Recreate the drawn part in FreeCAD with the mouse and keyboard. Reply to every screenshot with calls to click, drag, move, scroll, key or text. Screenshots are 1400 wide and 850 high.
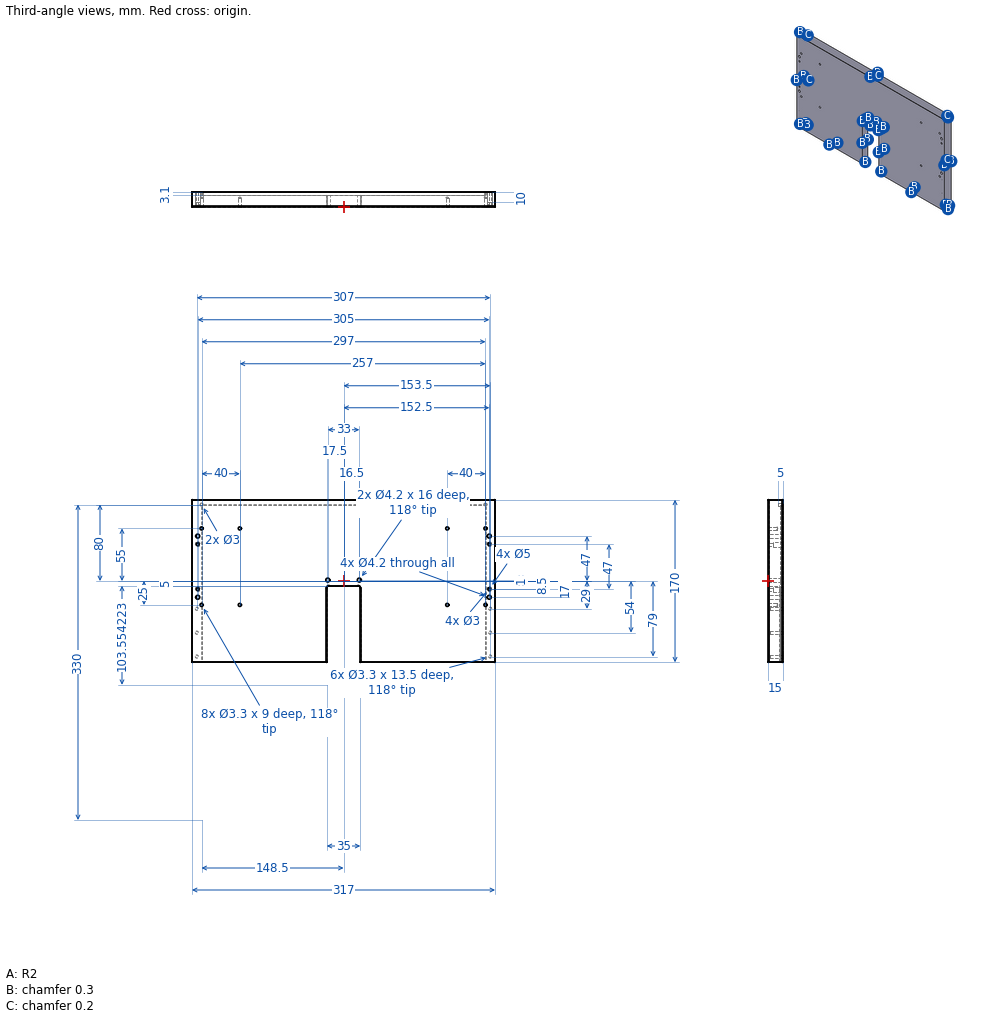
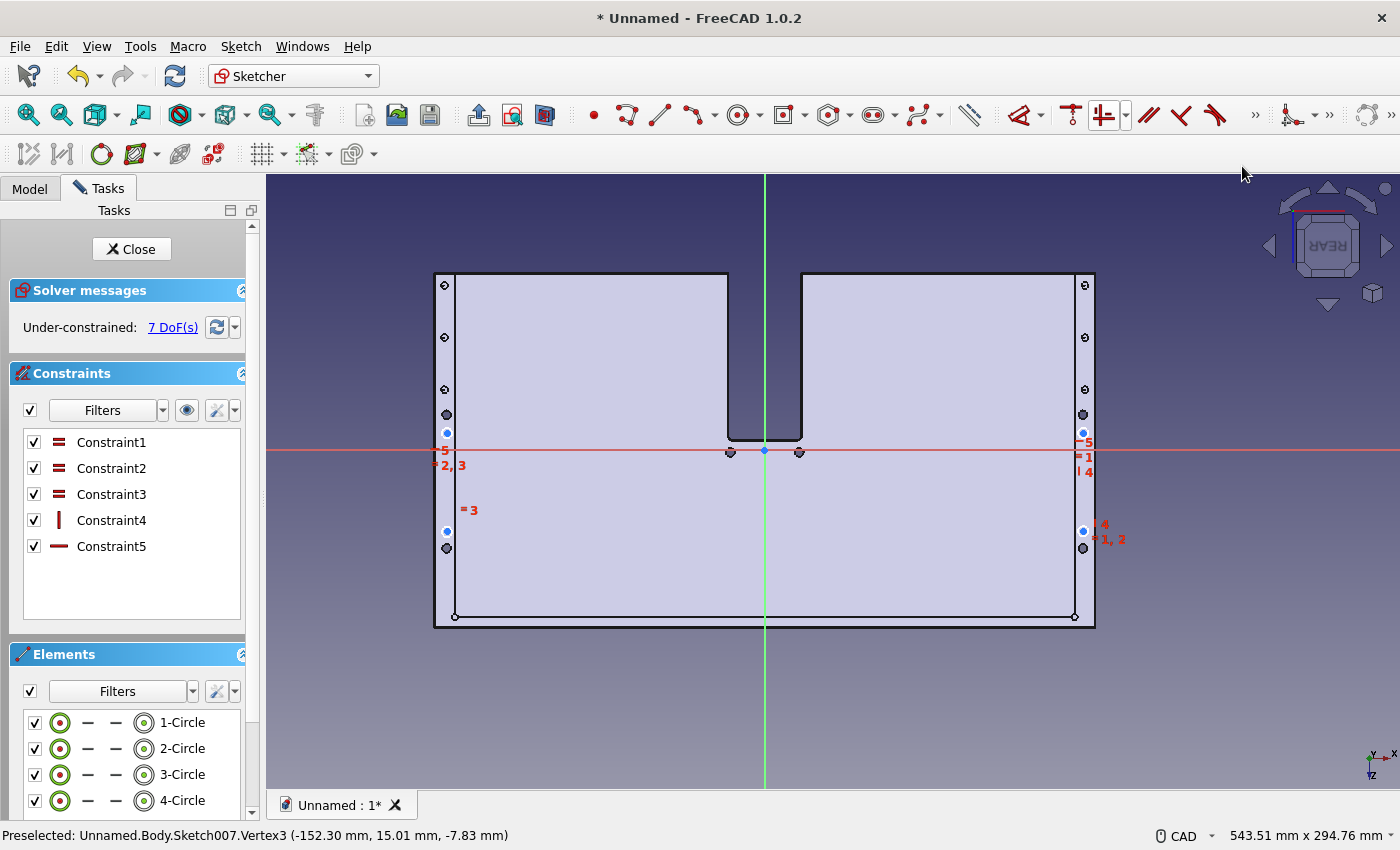
click(447, 433)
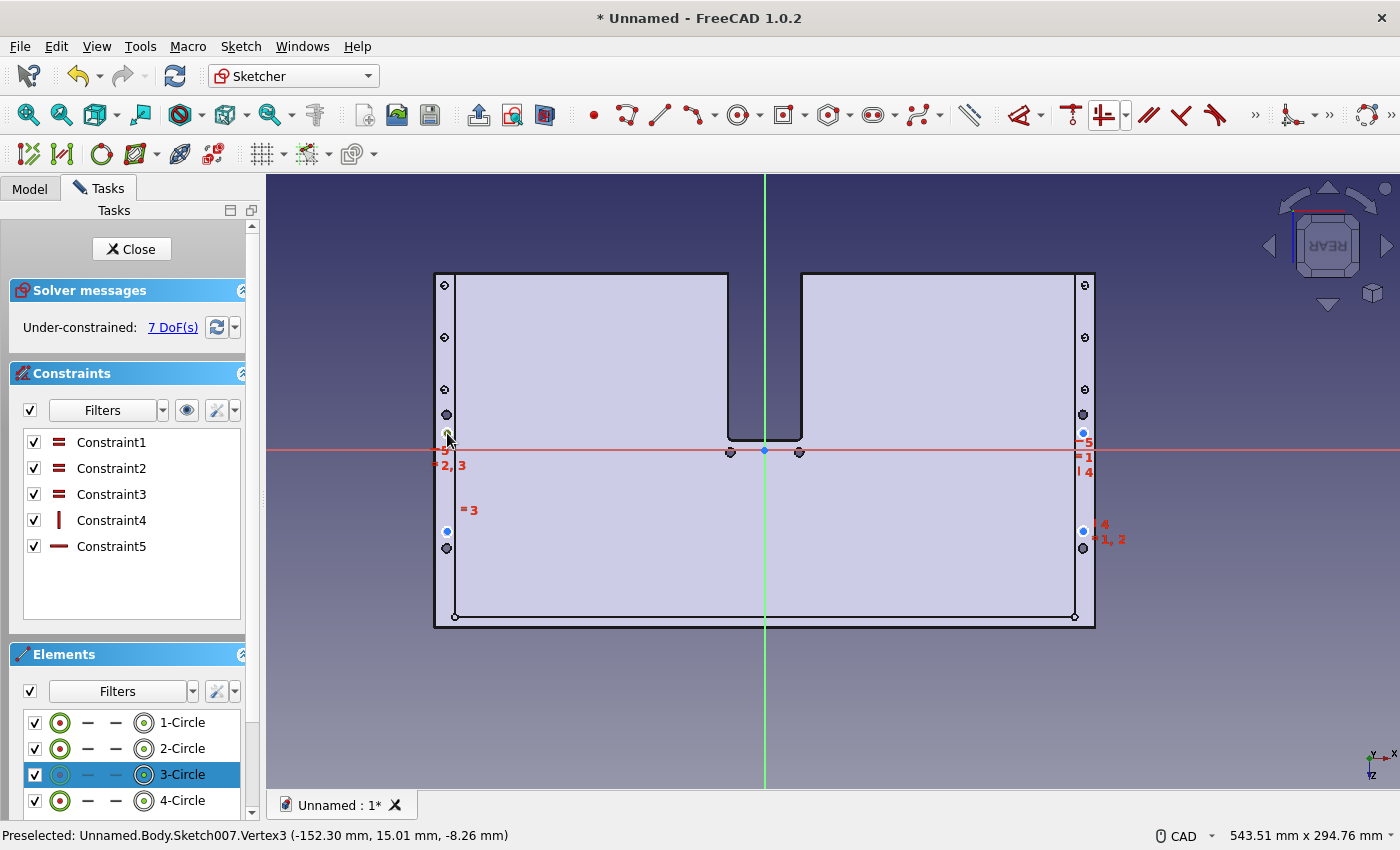
click(447, 532)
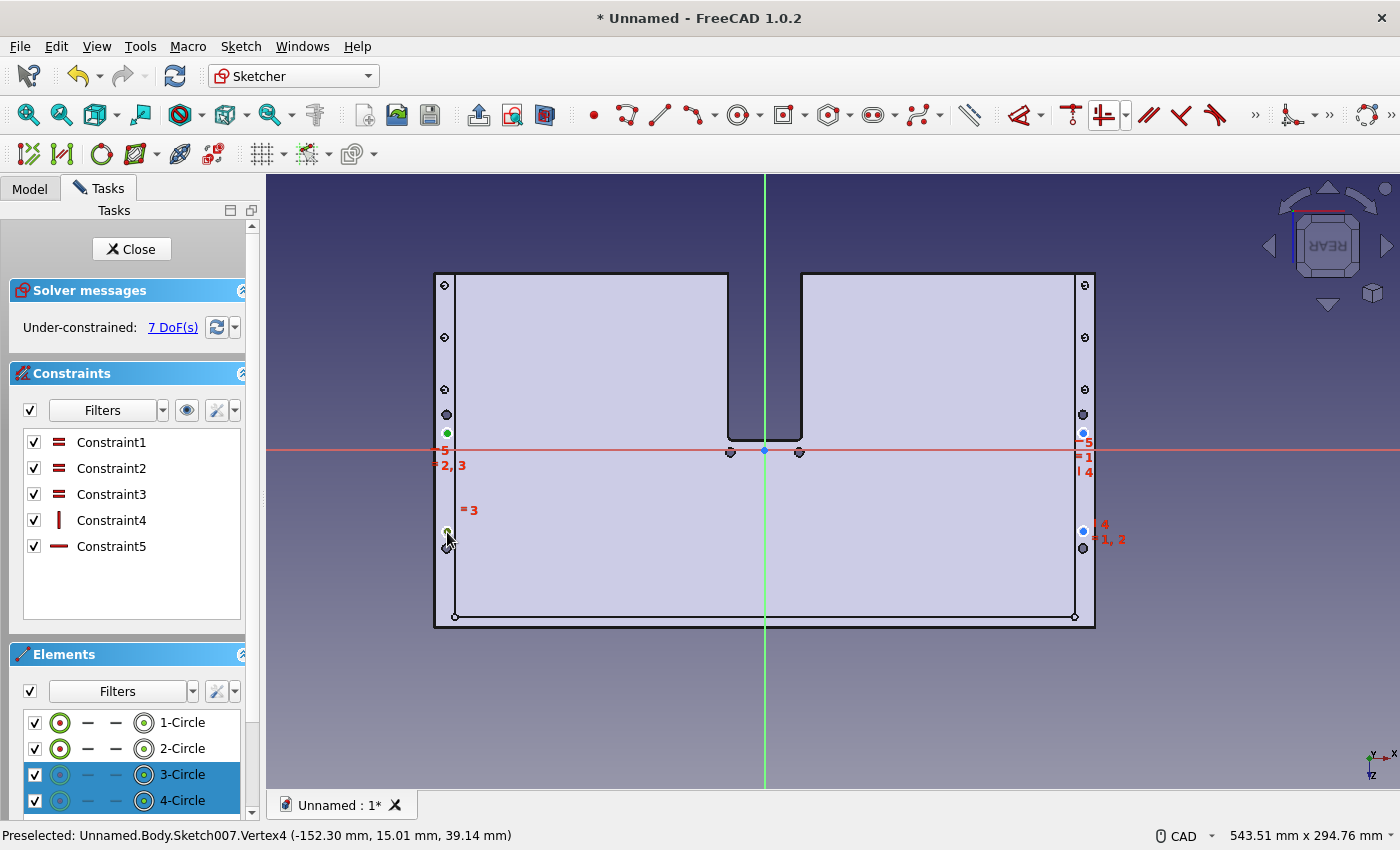
key(v)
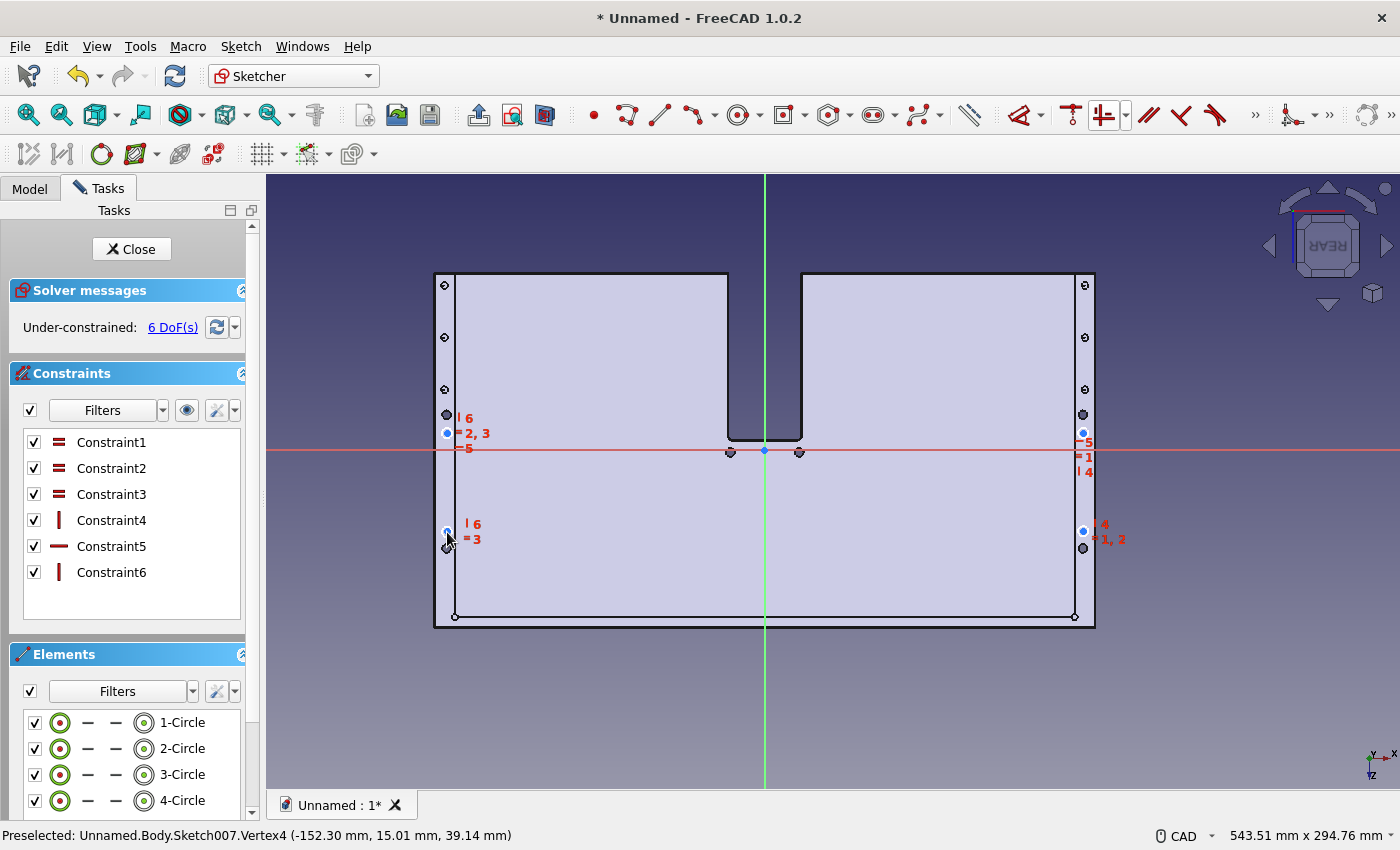
click(1083, 531)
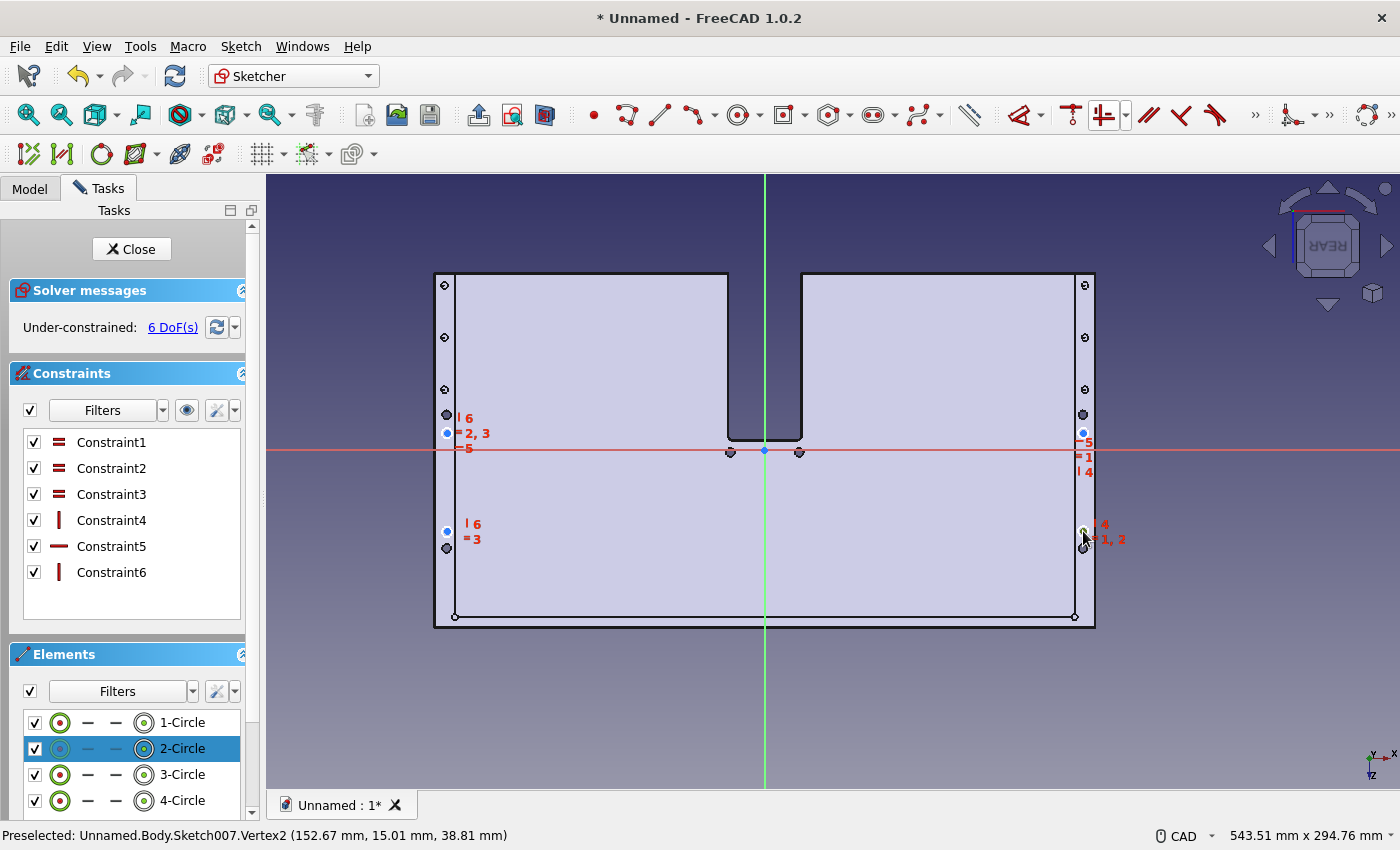
click(447, 532)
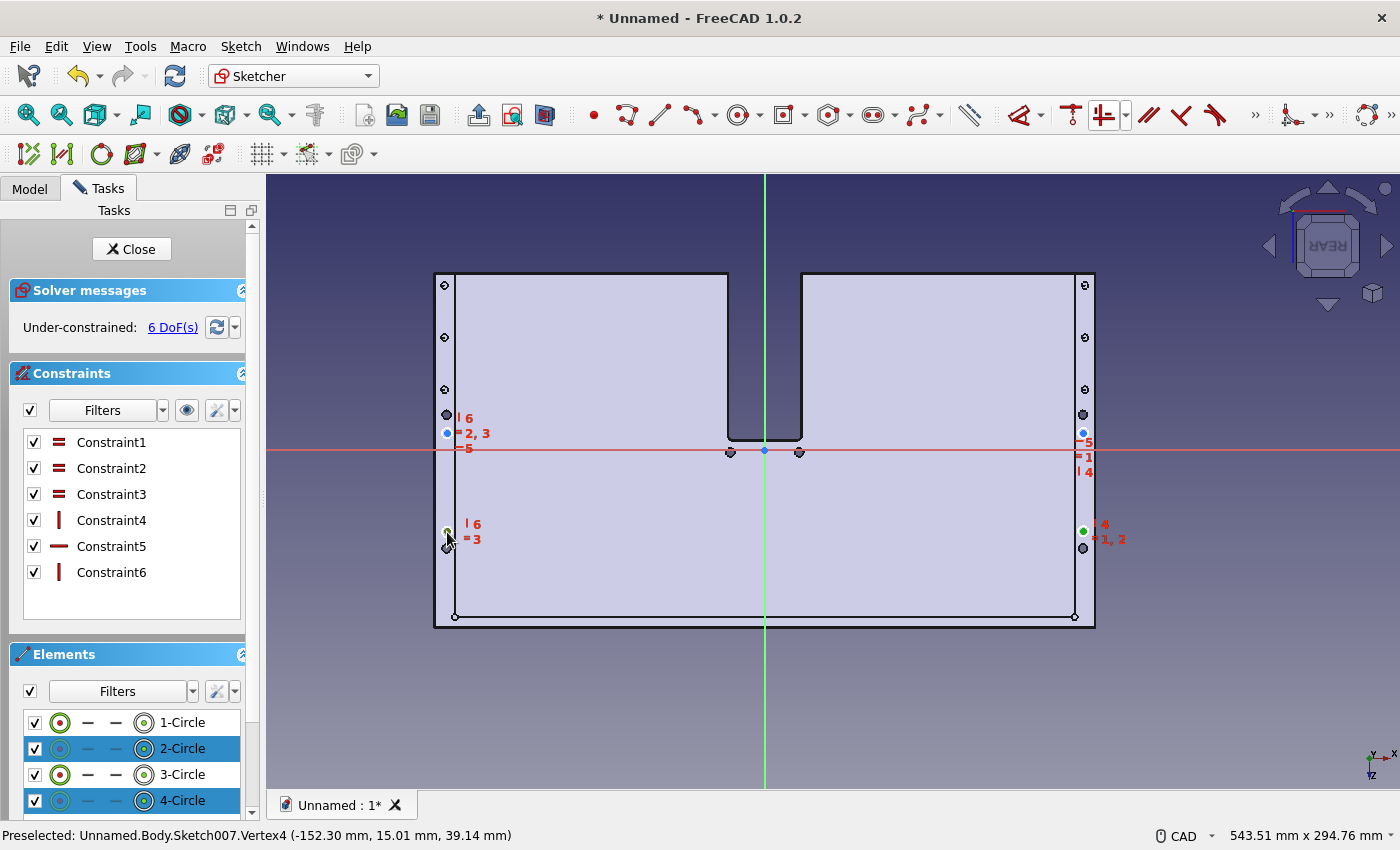
key(h)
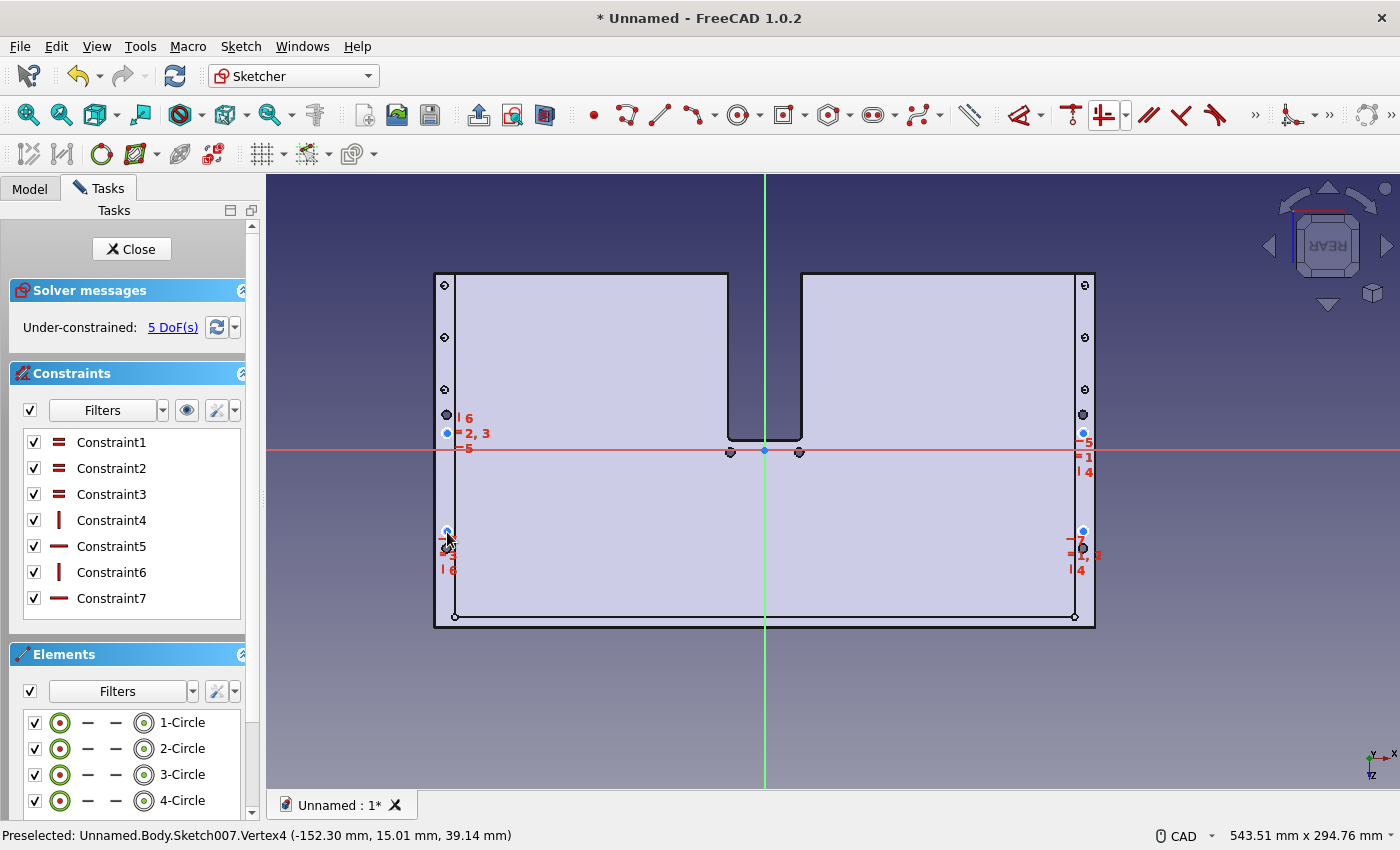
key(d)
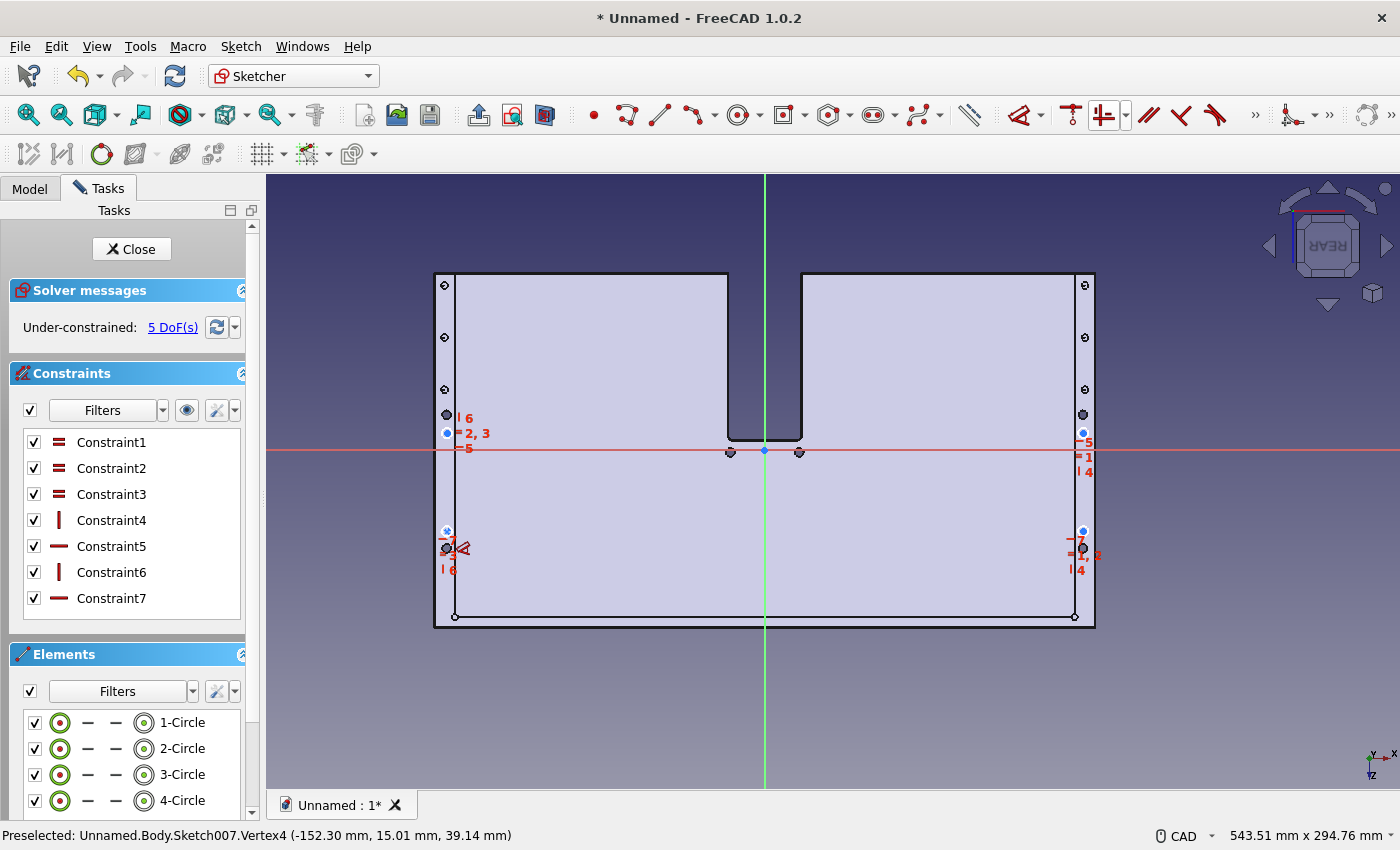
scroll(1078, 433, up, 7)